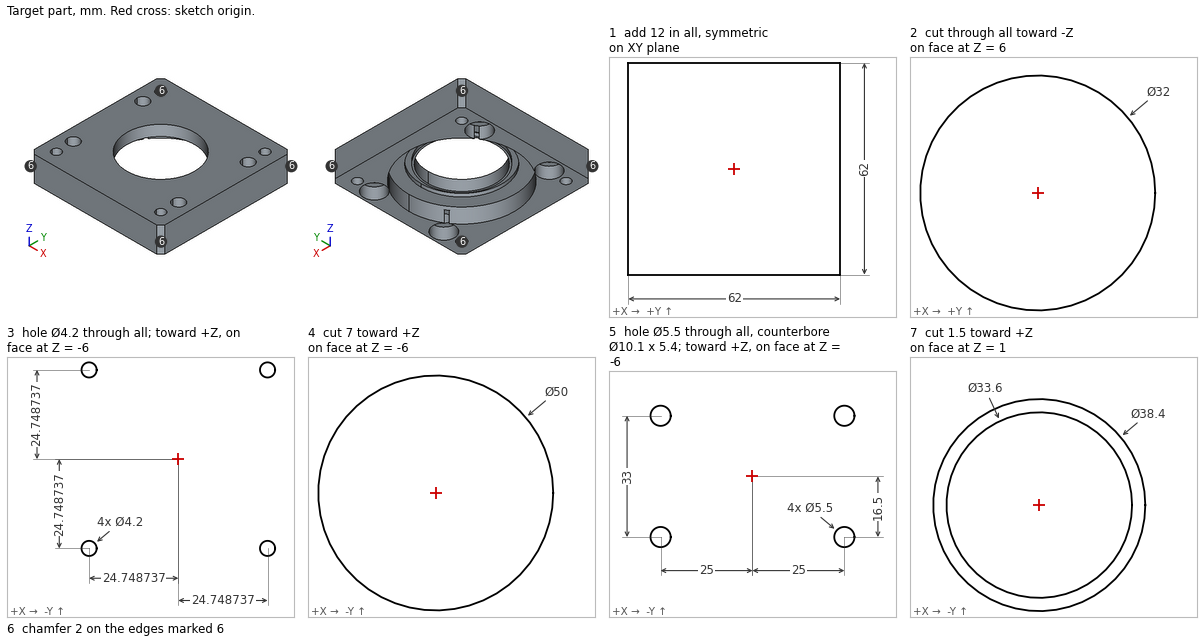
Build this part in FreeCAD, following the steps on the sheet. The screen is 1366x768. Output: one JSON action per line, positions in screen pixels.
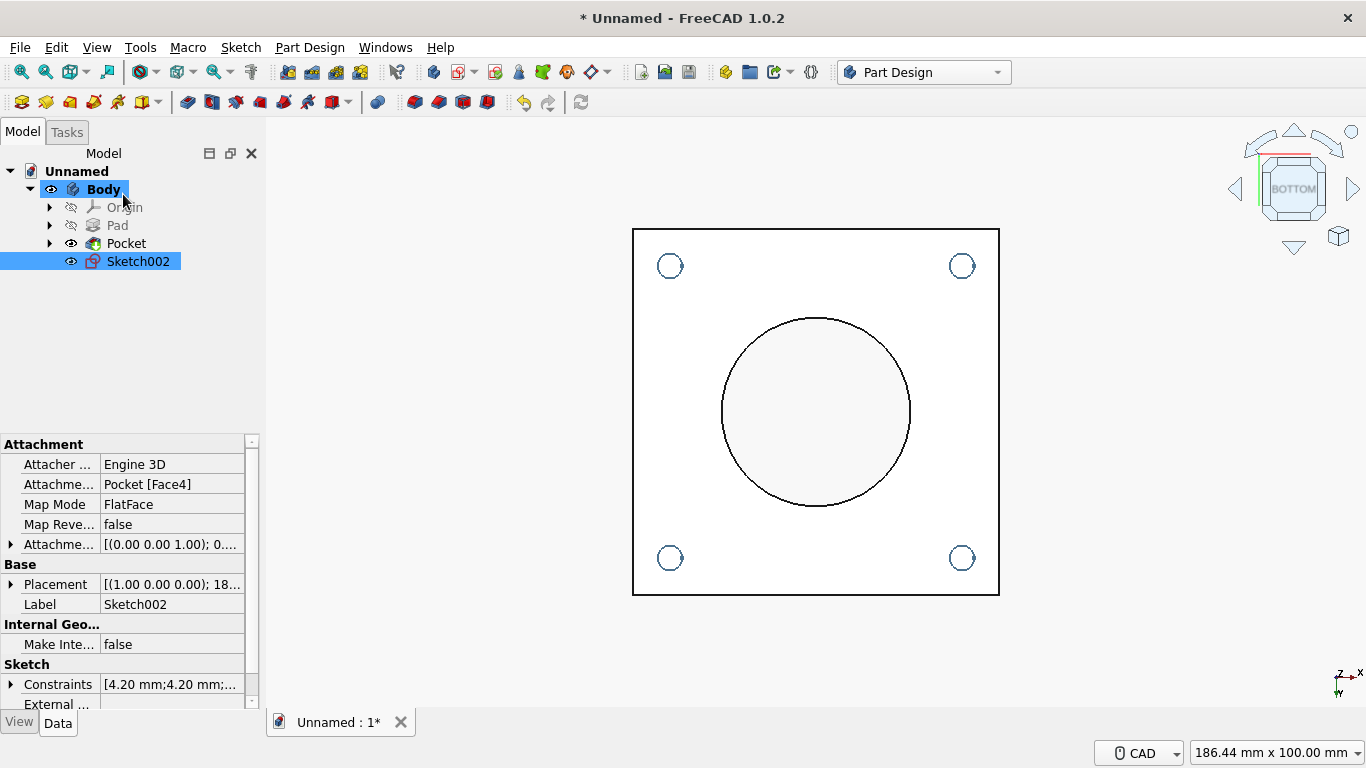
{"action": "left_click", "coordinate": [212, 102]}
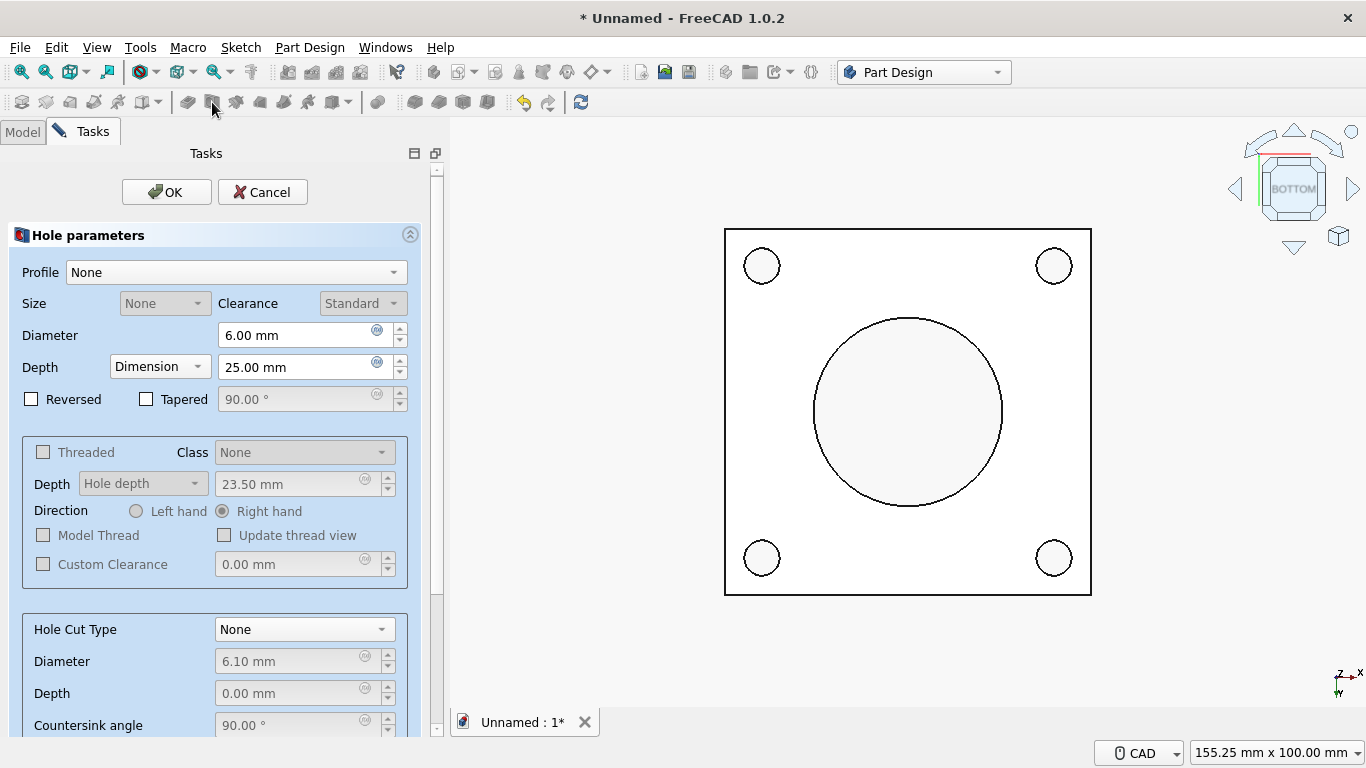
{"action": "triple_click", "coordinate": [305, 335]}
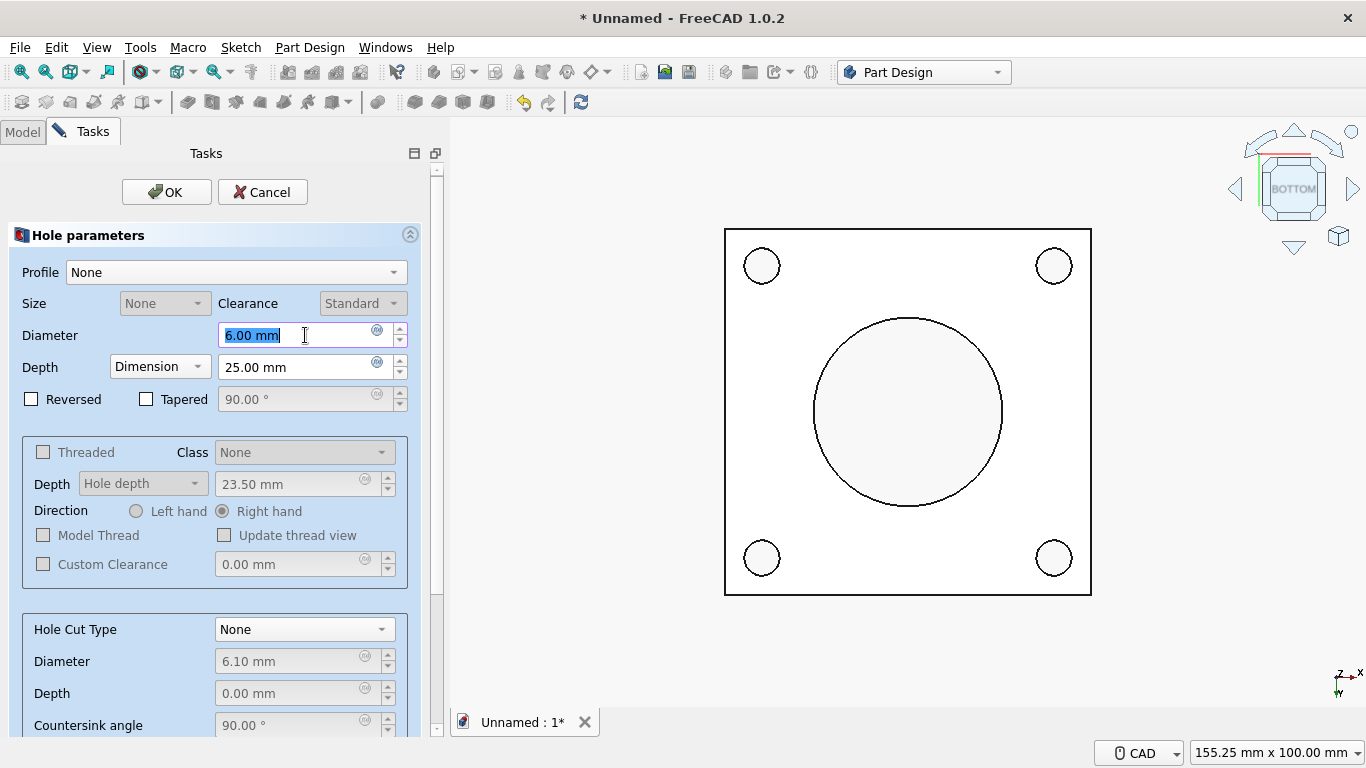
{"action": "type", "text": "4.2"}
{"action": "key", "text": "Tab"}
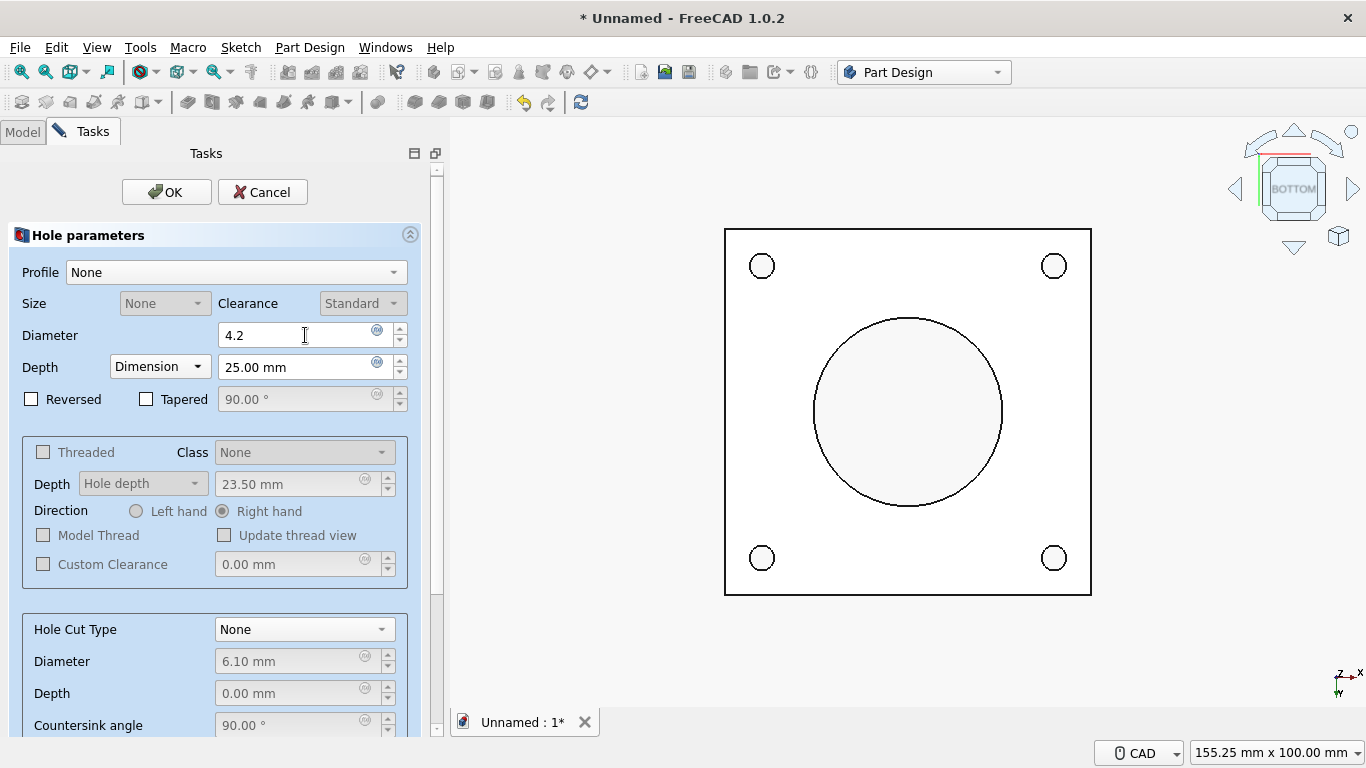
{"action": "left_click", "coordinate": [161, 366]}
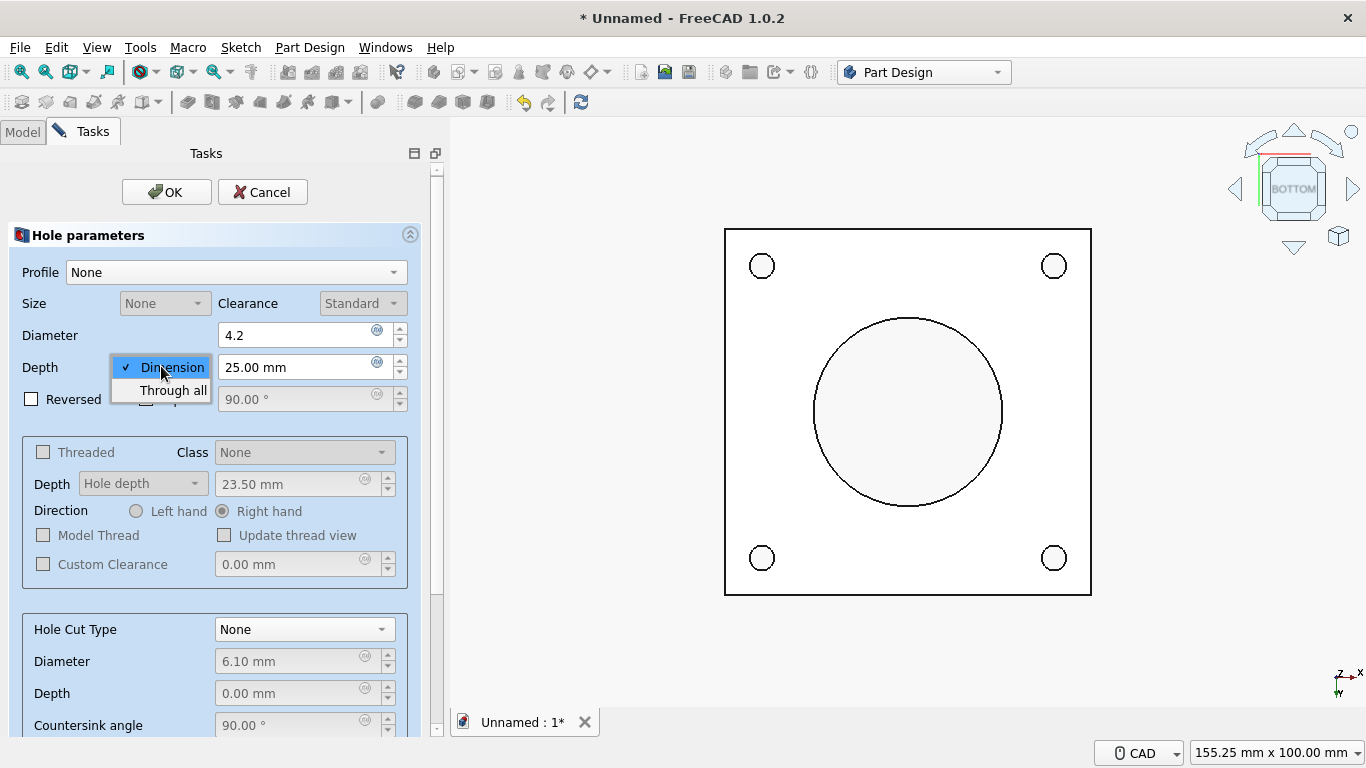
{"action": "left_click", "coordinate": [160, 390]}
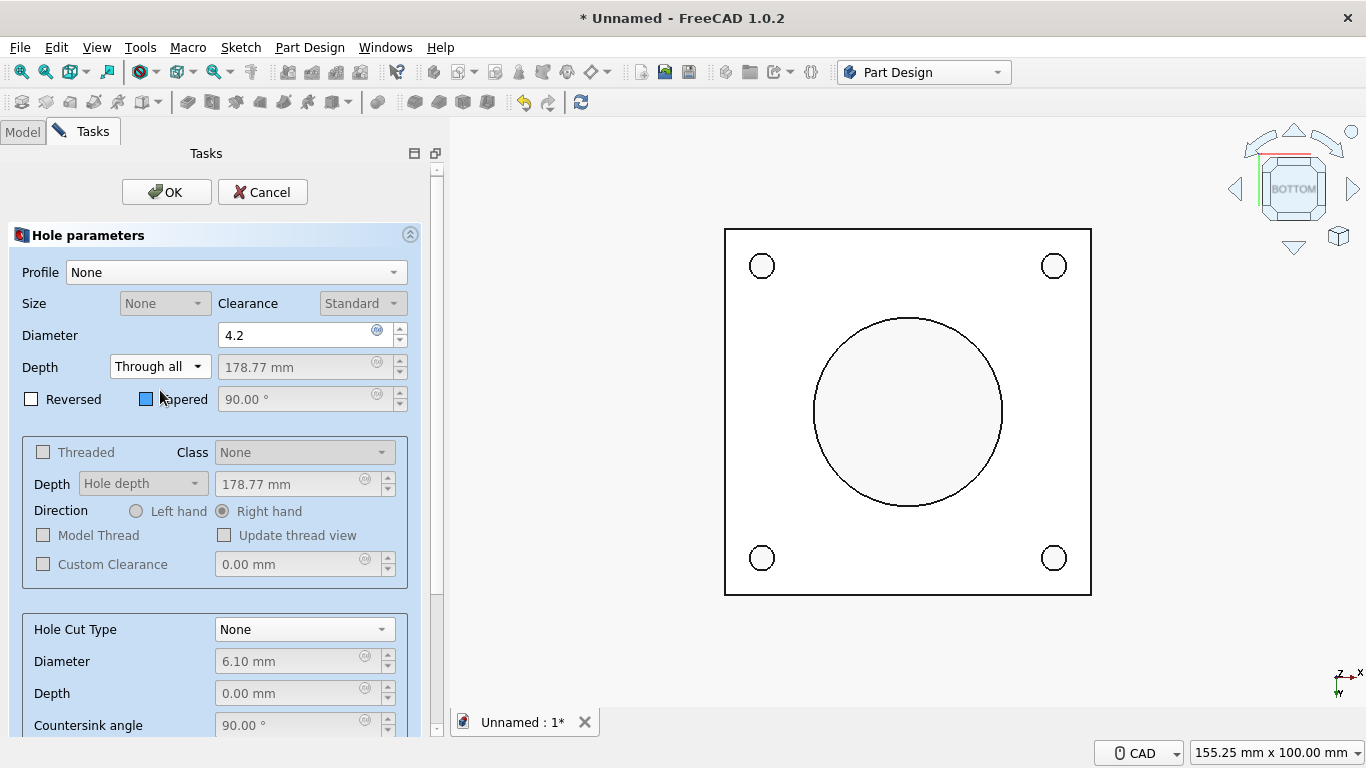
{"action": "left_click", "coordinate": [167, 192]}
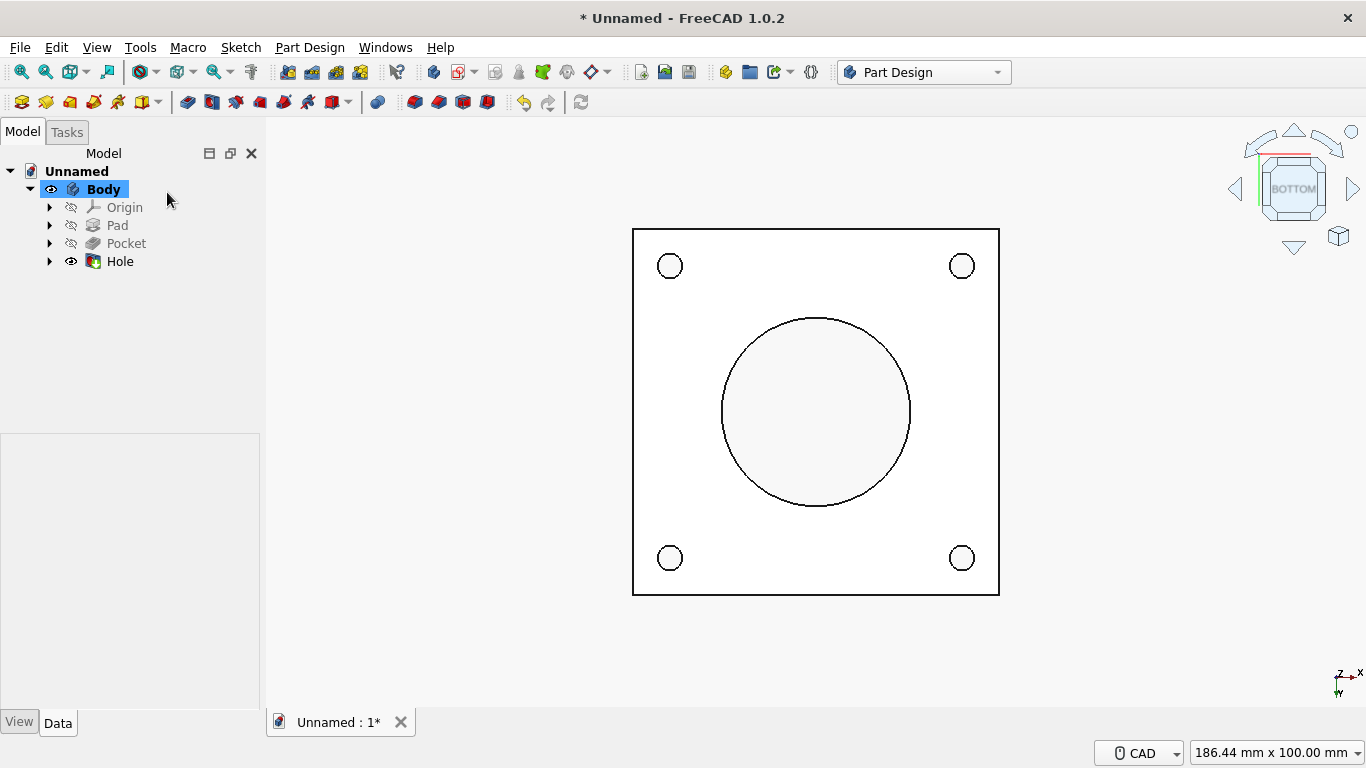
{"action": "left_click", "coordinate": [921, 516]}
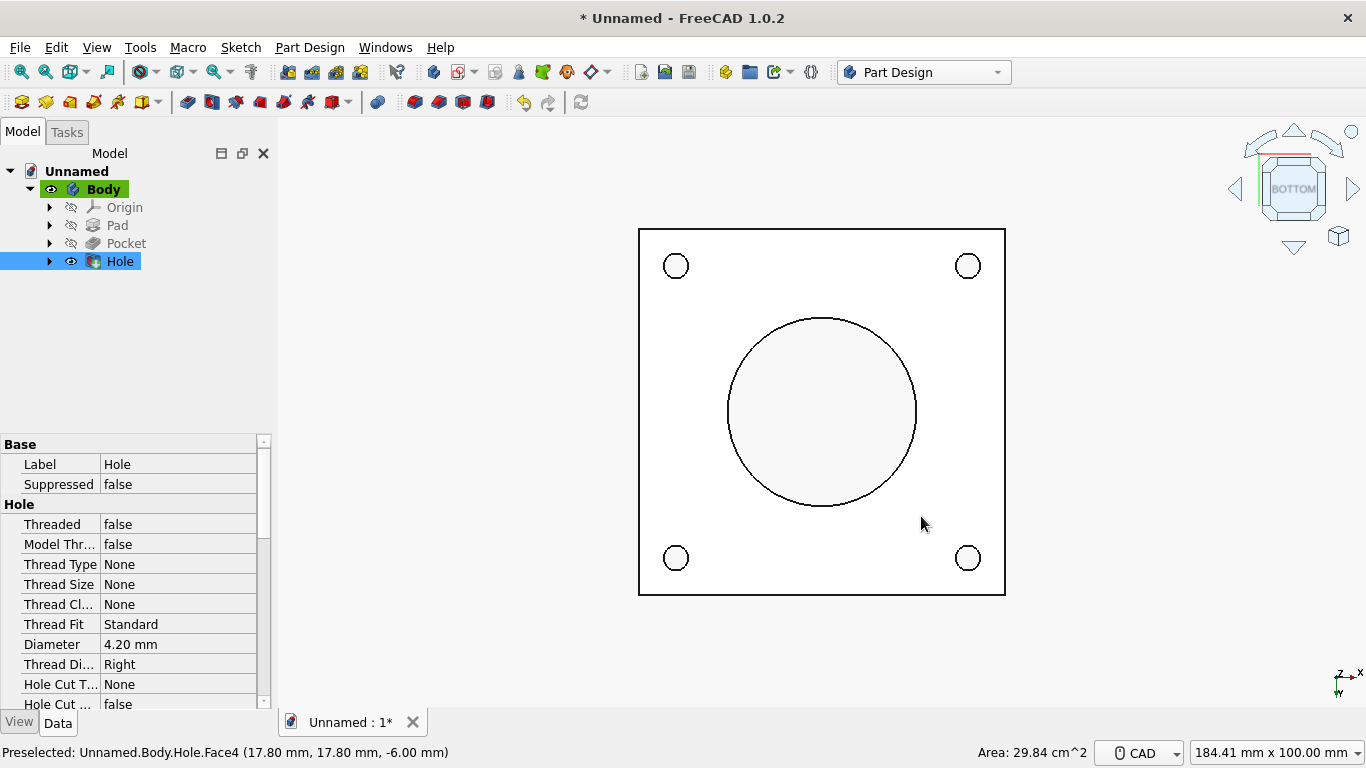
{"action": "left_click", "coordinate": [458, 72]}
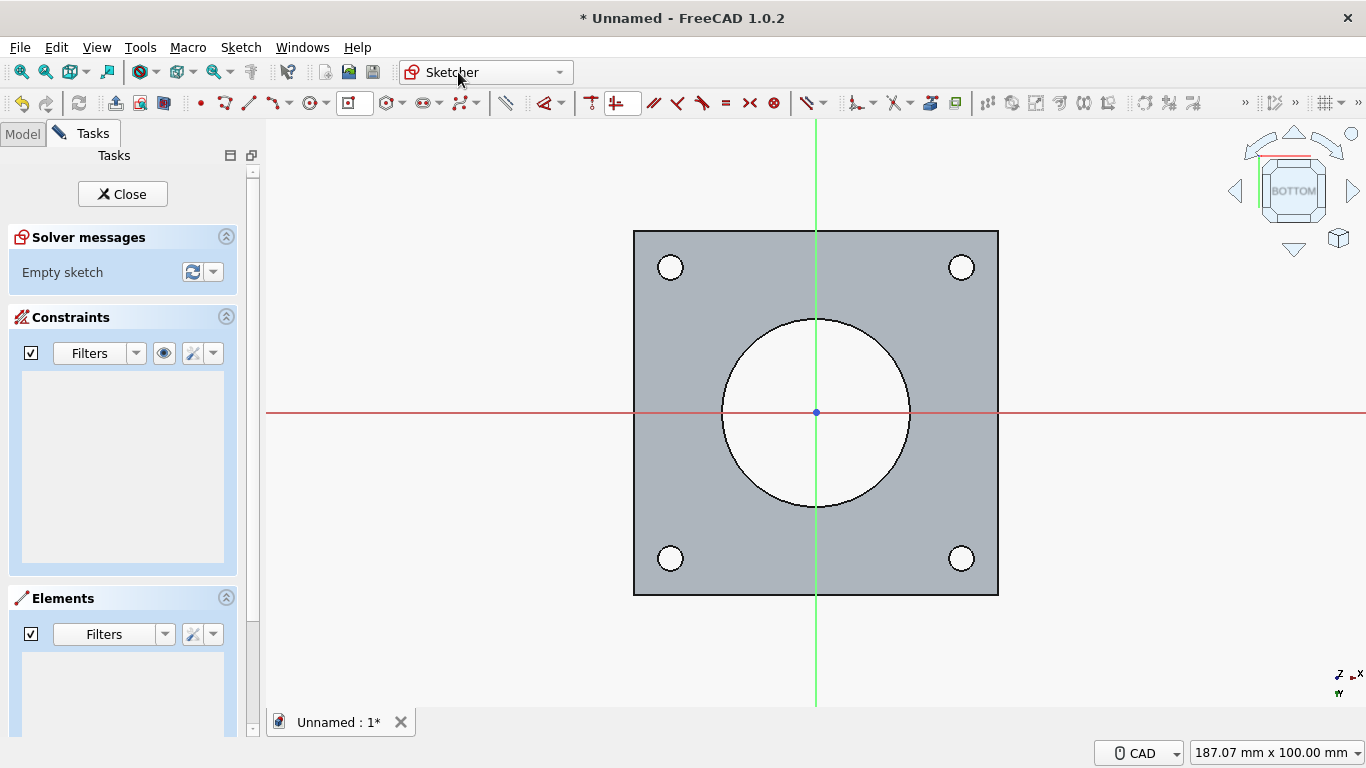
{"action": "left_click", "coordinate": [310, 104]}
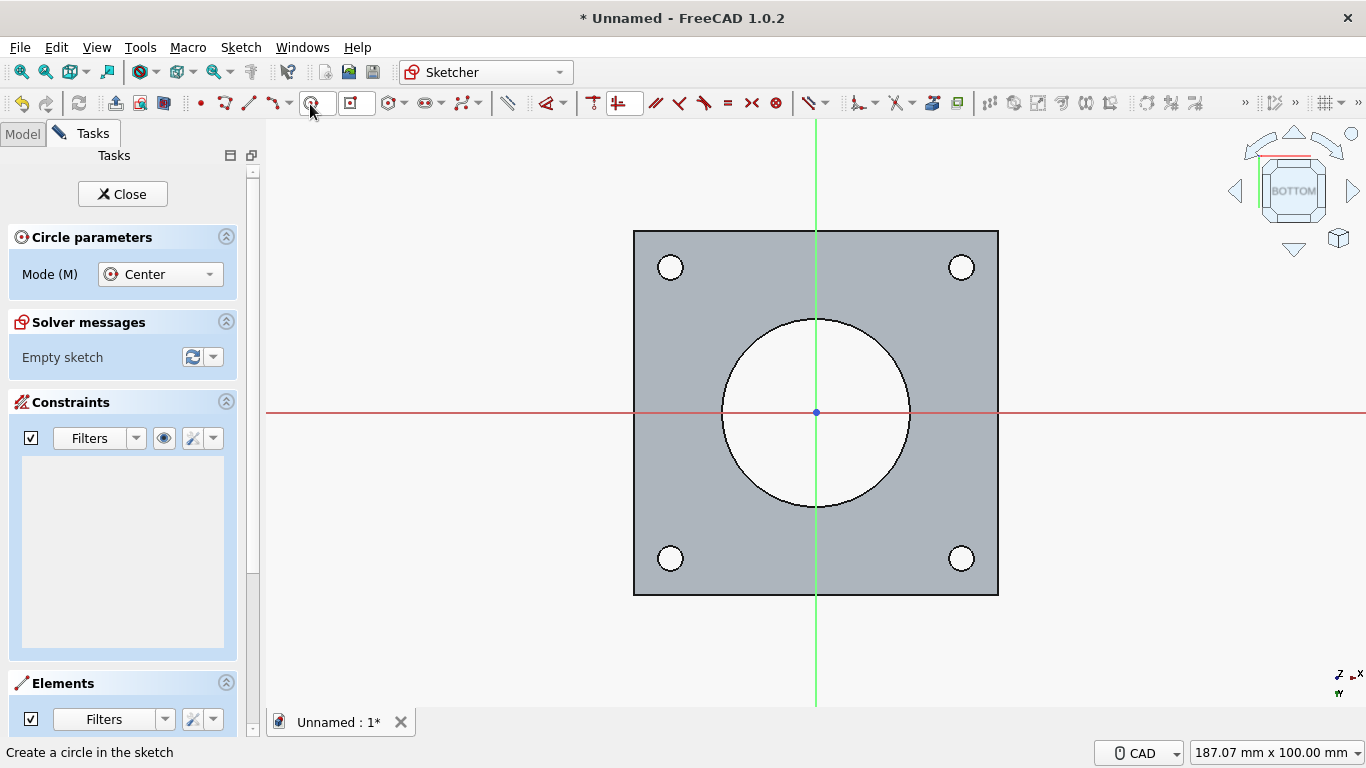
{"action": "left_click", "coordinate": [816, 413]}
{"action": "mouse_move", "coordinate": [920, 309]}